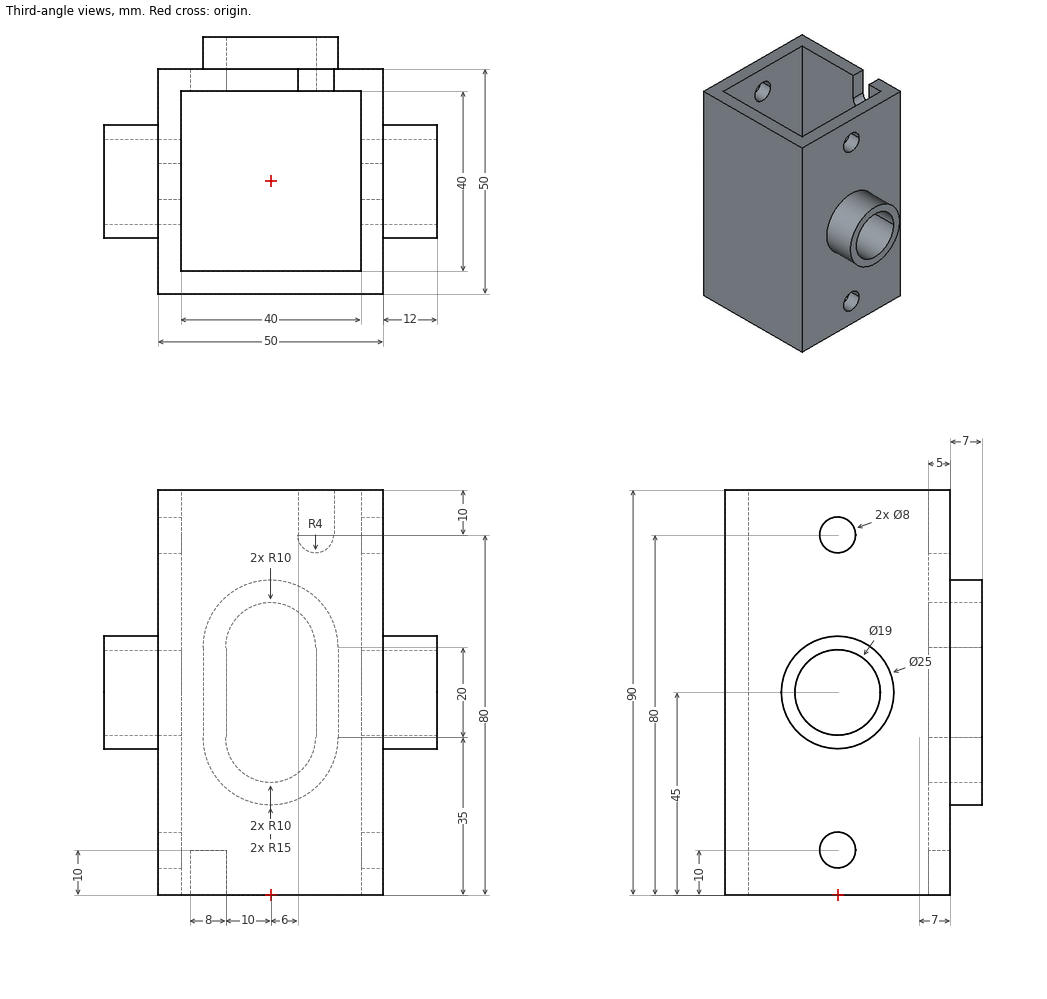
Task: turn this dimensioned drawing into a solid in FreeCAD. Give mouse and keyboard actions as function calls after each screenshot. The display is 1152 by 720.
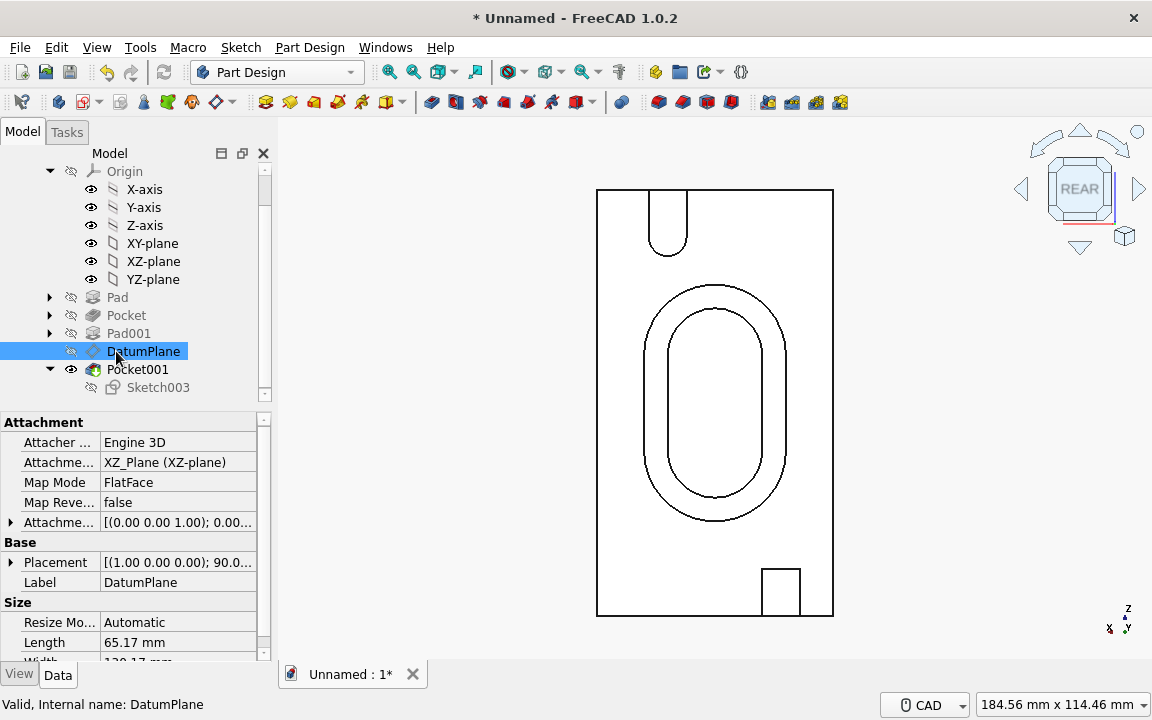
key(0)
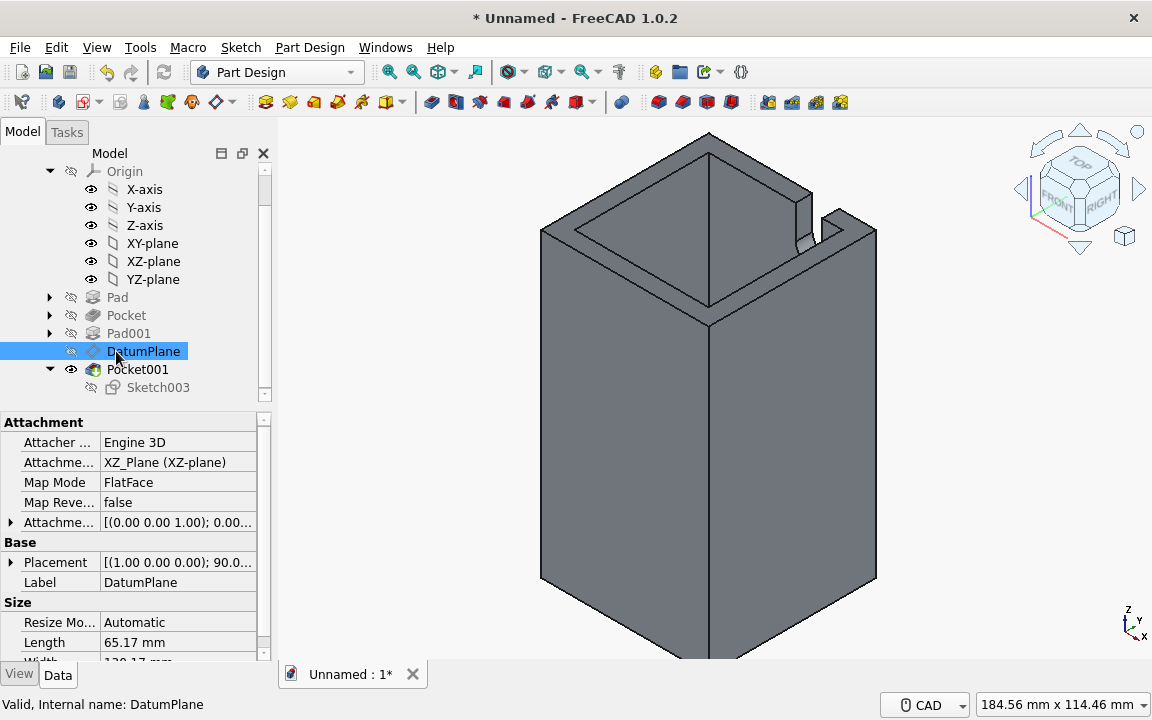
key(v)
key(f)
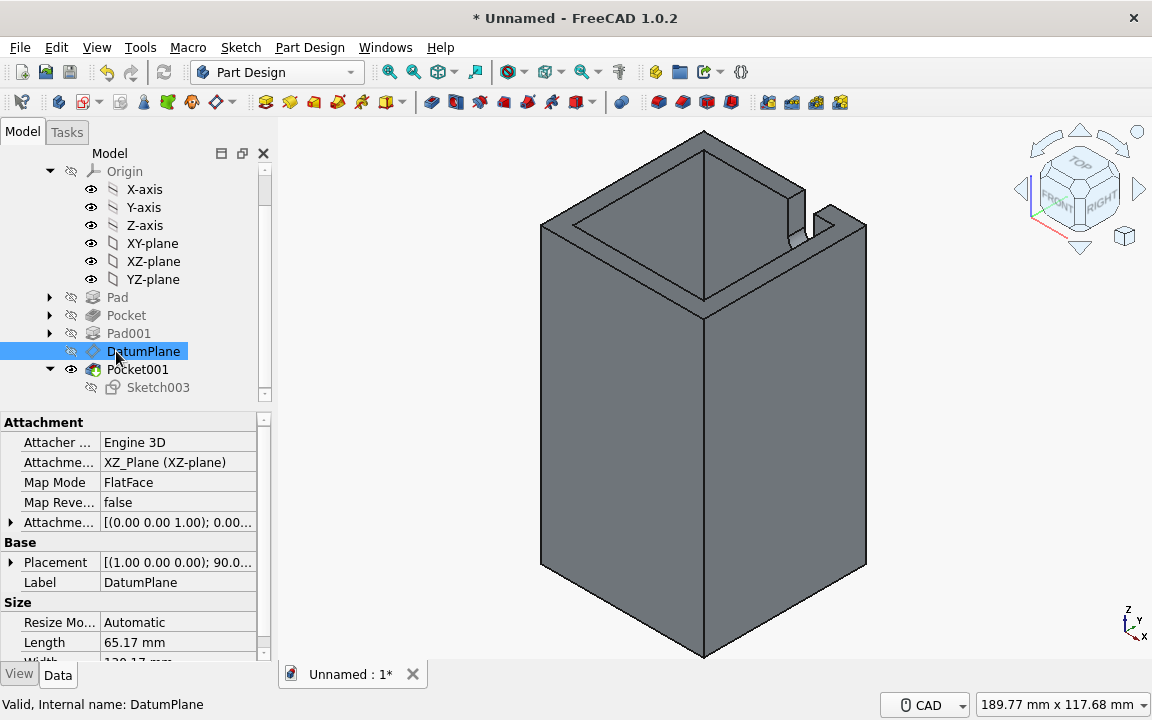
click(785, 392)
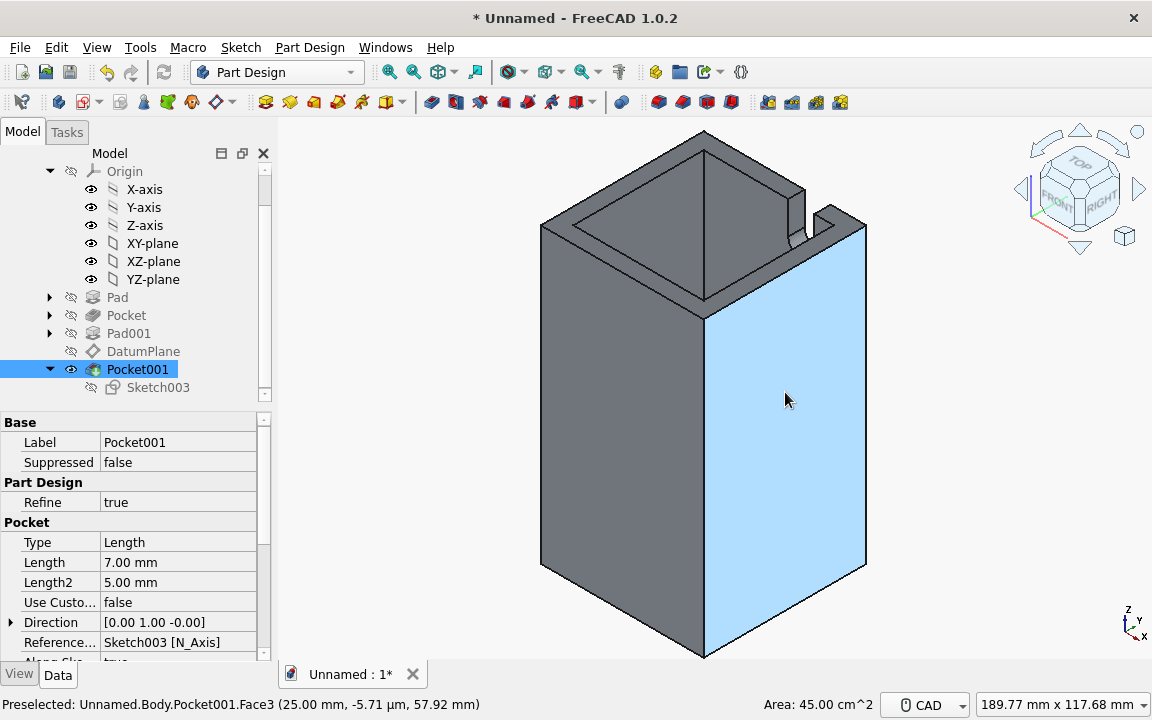
click(84, 102)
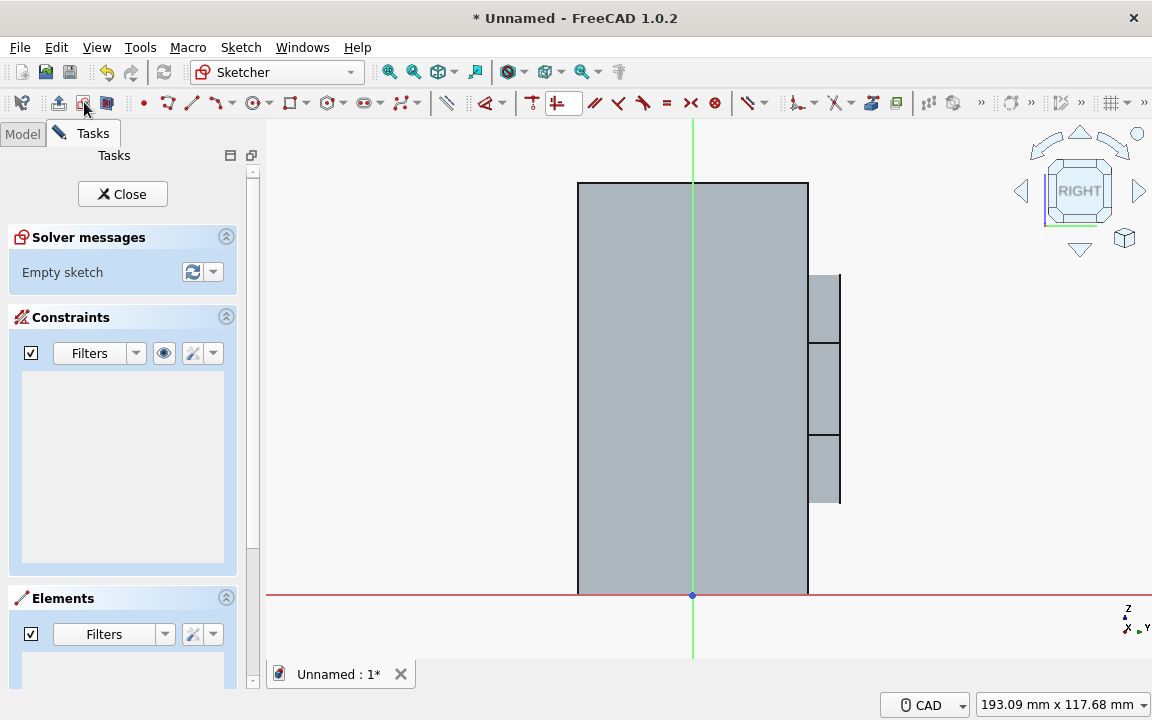
click(254, 104)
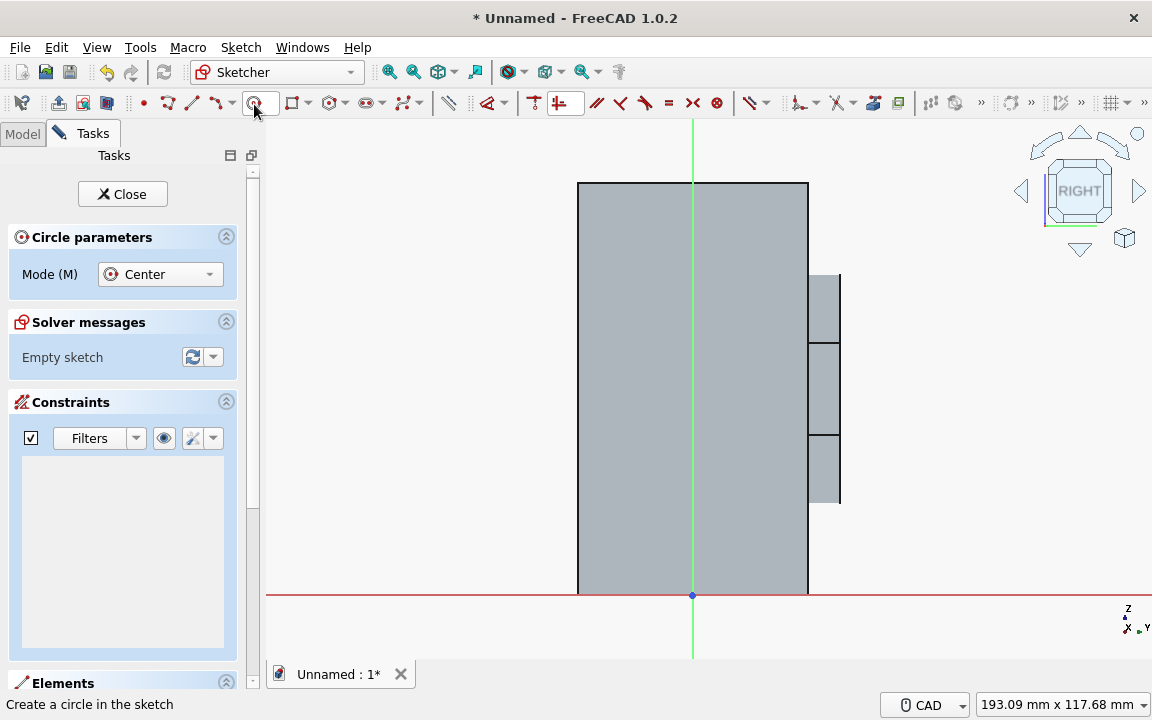
click(693, 389)
click(733, 348)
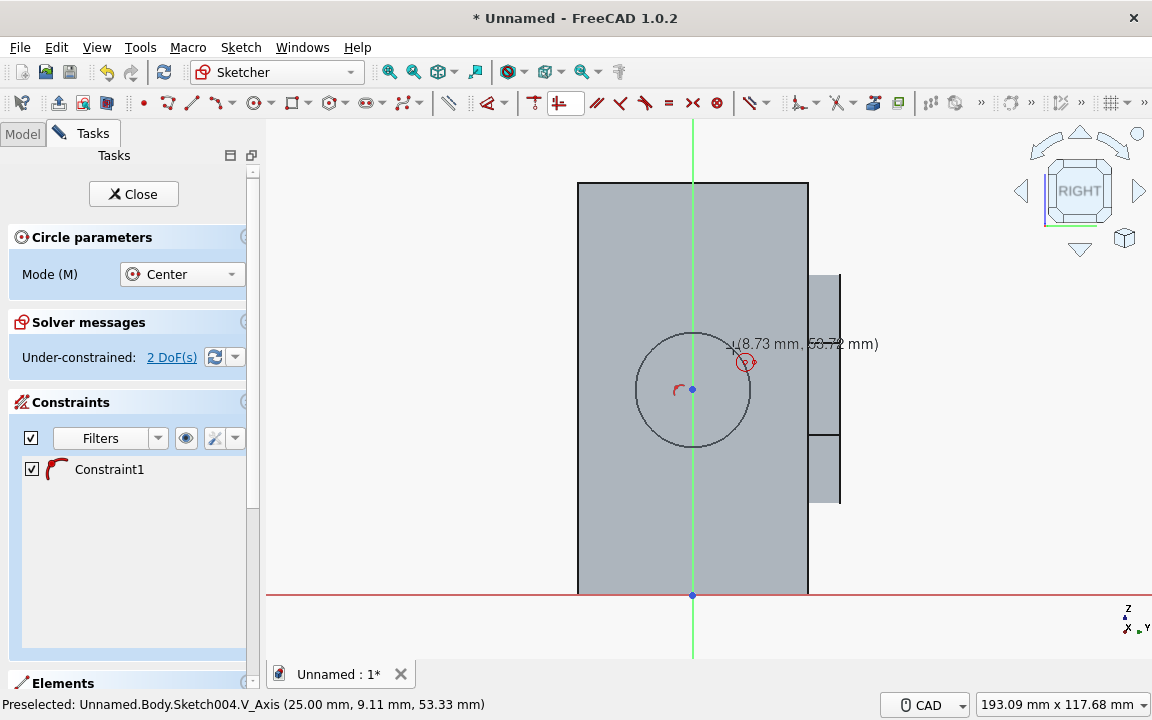
click(693, 390)
click(724, 358)
key(Escape)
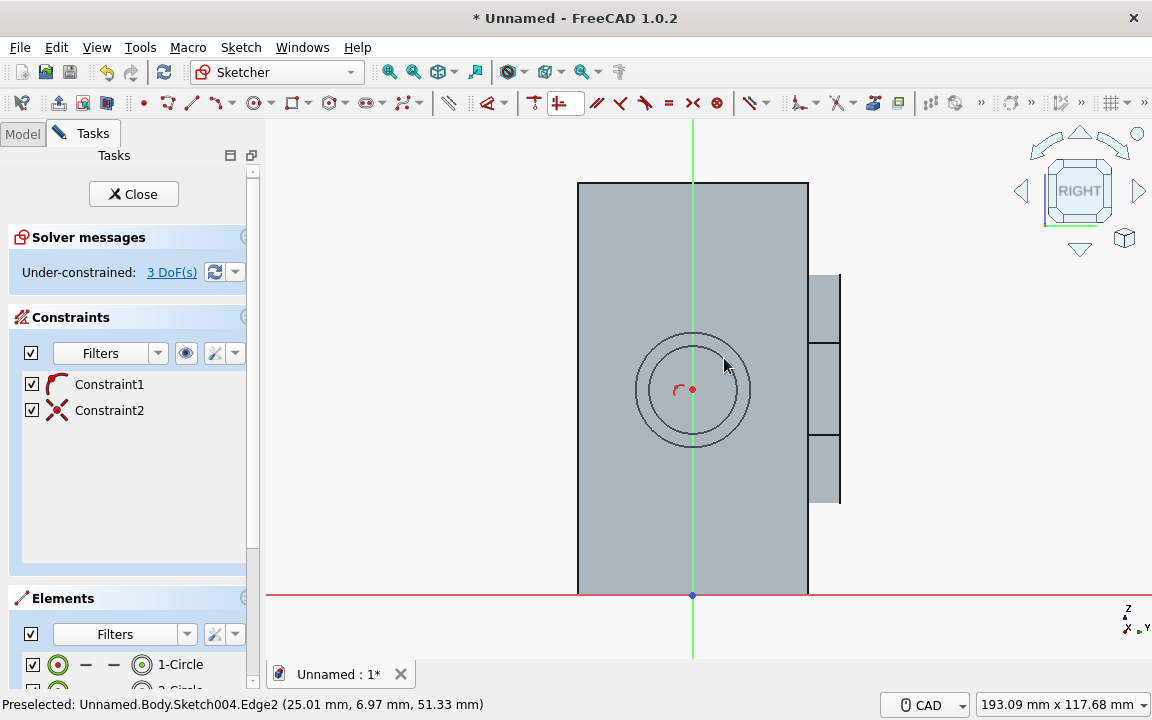
key(d)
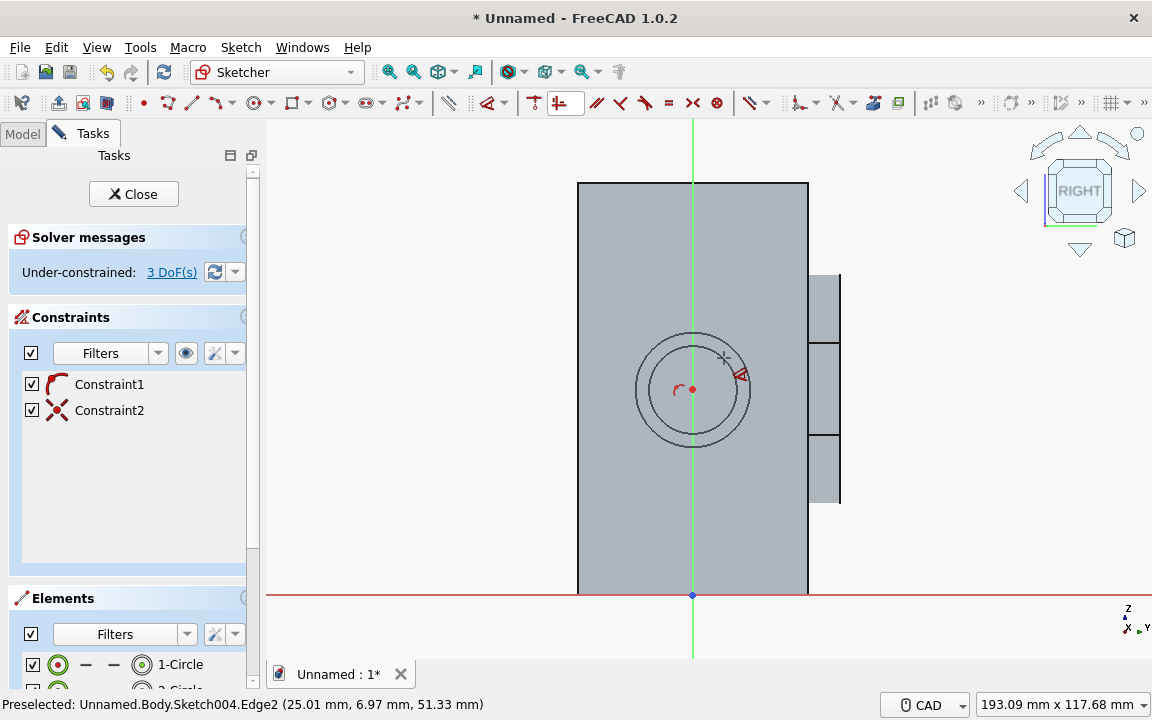
click(733, 349)
click(755, 326)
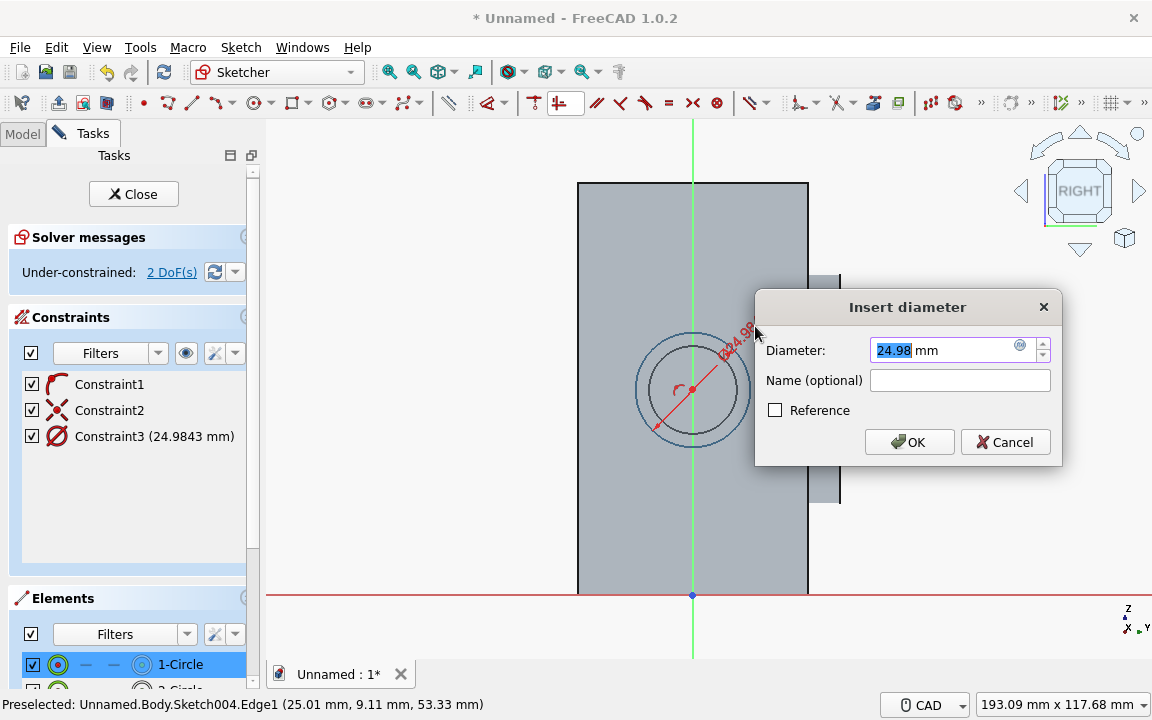
text(25)
key(Return)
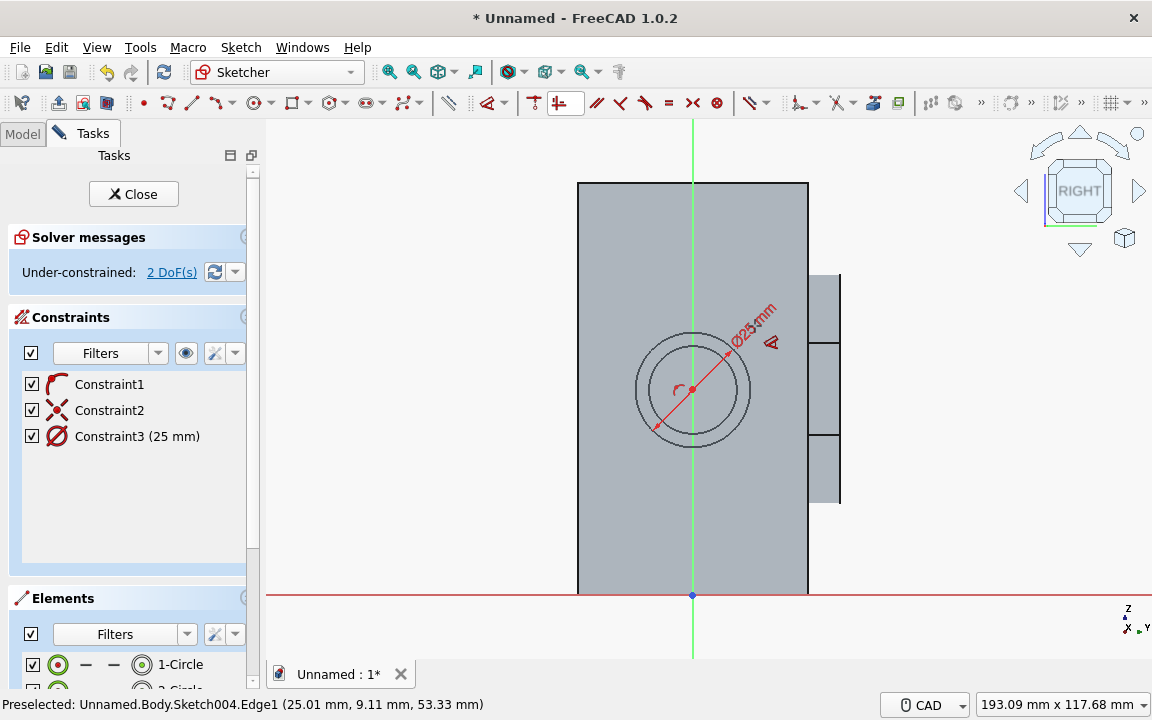
click(724, 359)
click(766, 369)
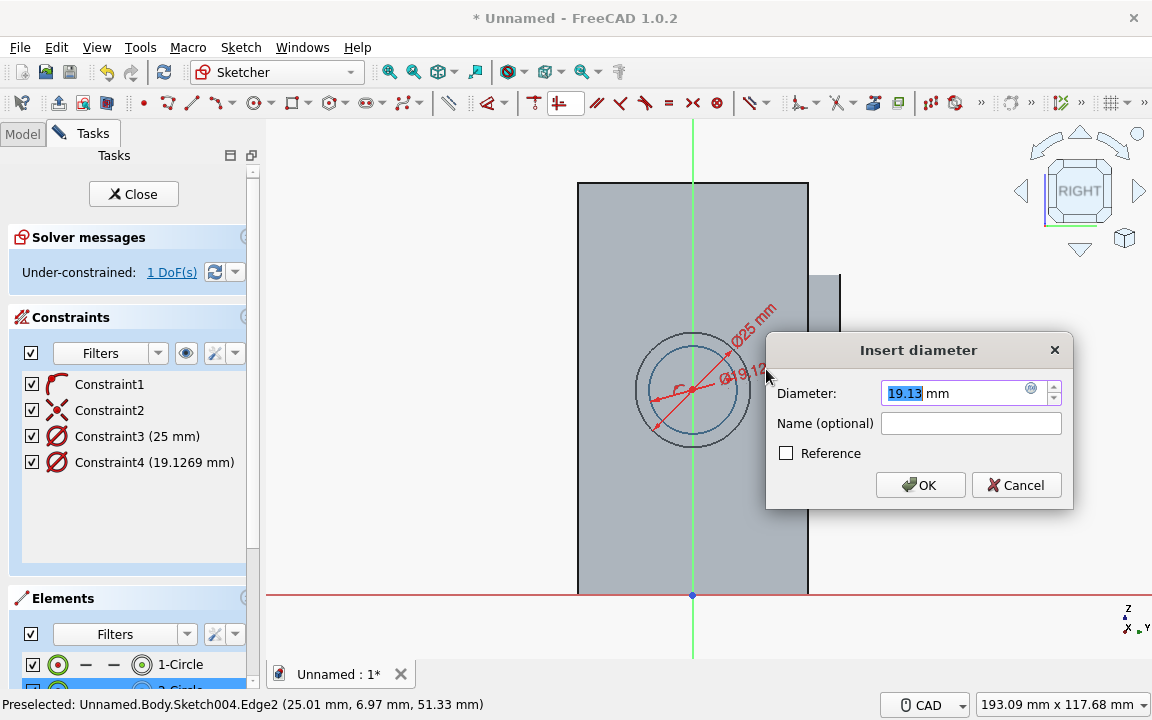
text(19)
key(Return)